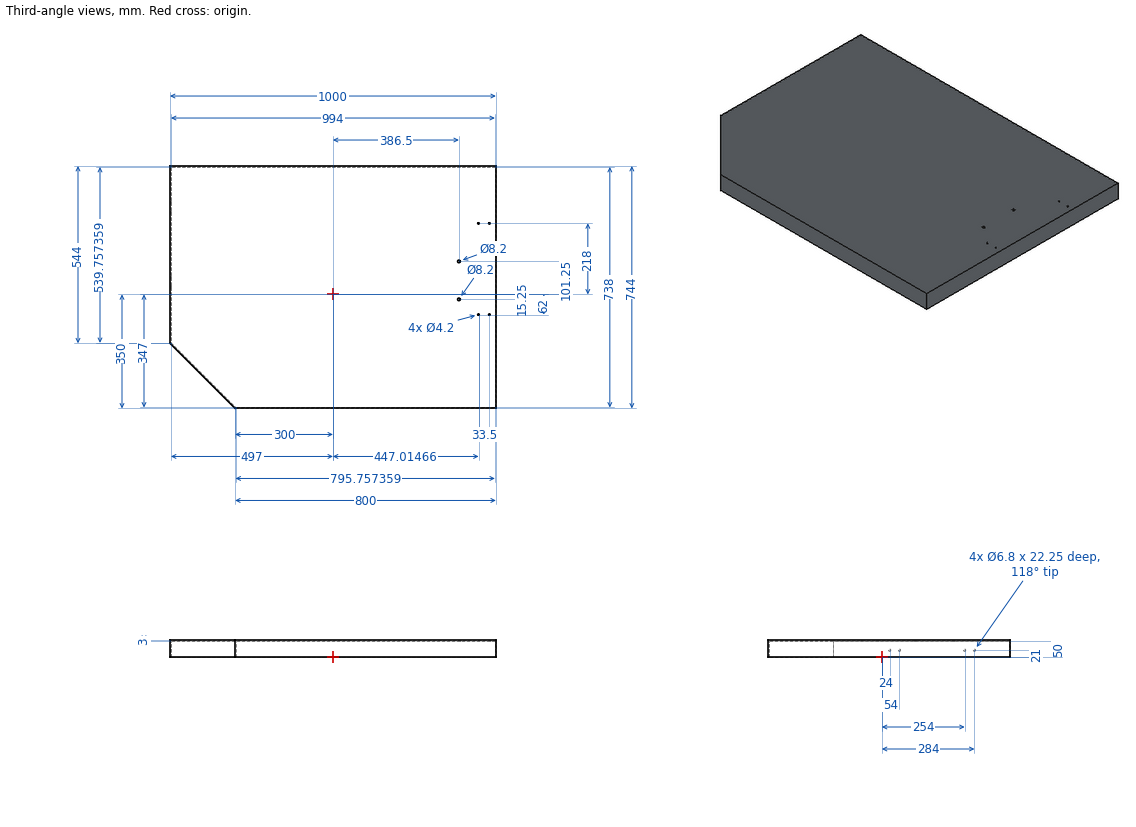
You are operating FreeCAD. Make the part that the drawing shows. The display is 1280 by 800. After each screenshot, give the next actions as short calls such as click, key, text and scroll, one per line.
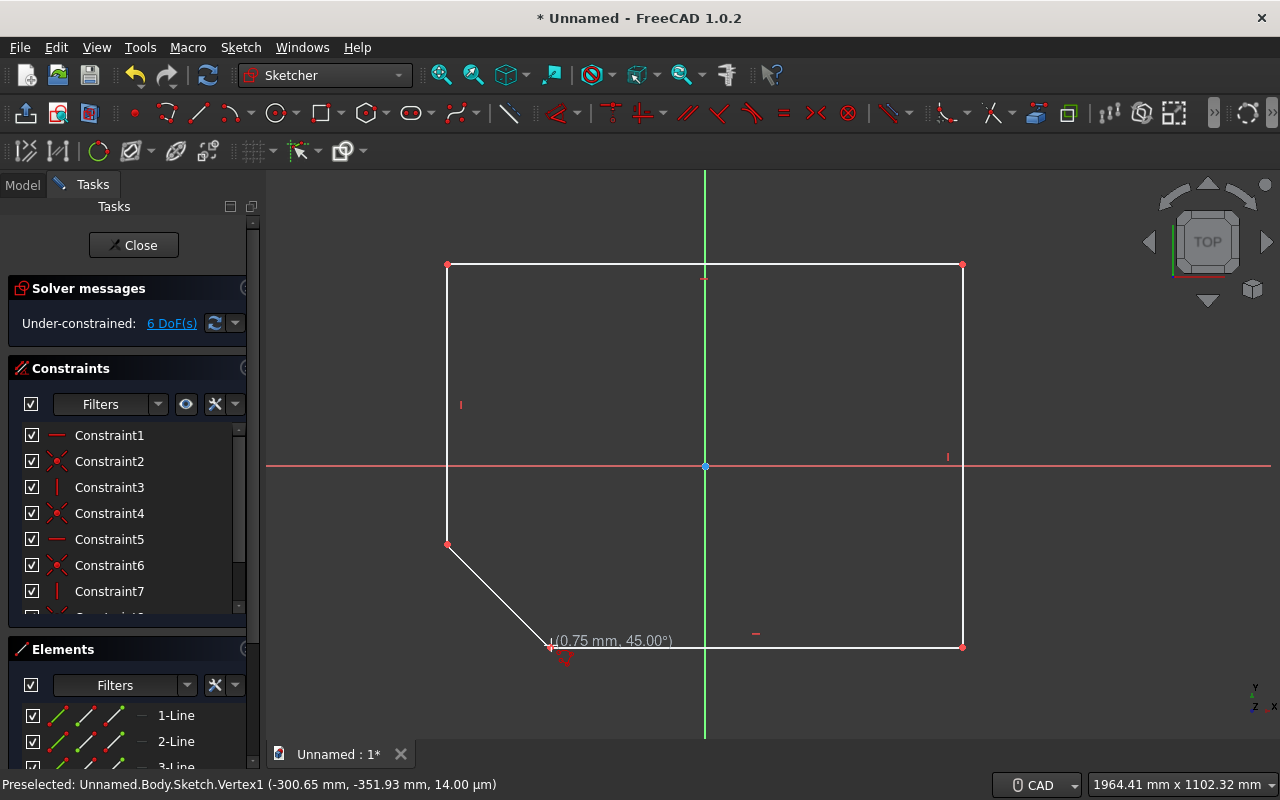
scroll(449, 543, up, 12)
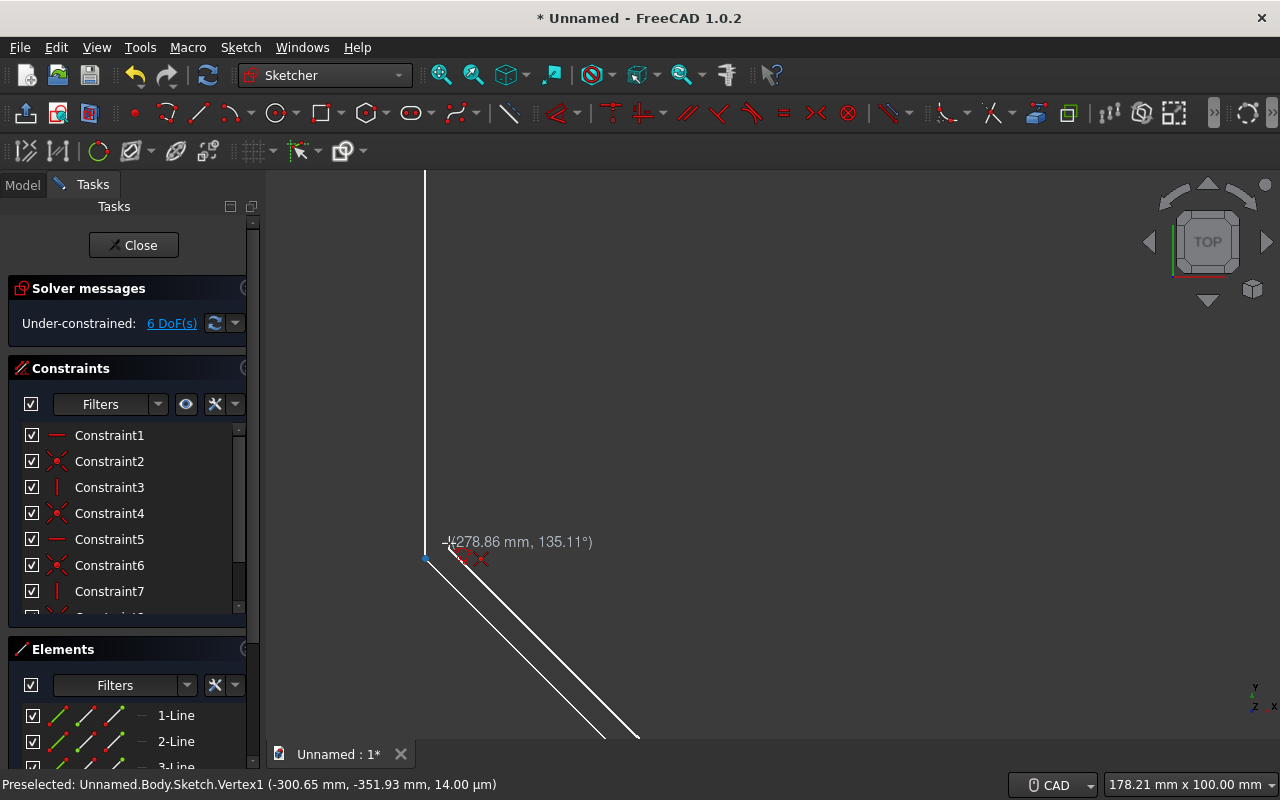
click(443, 538)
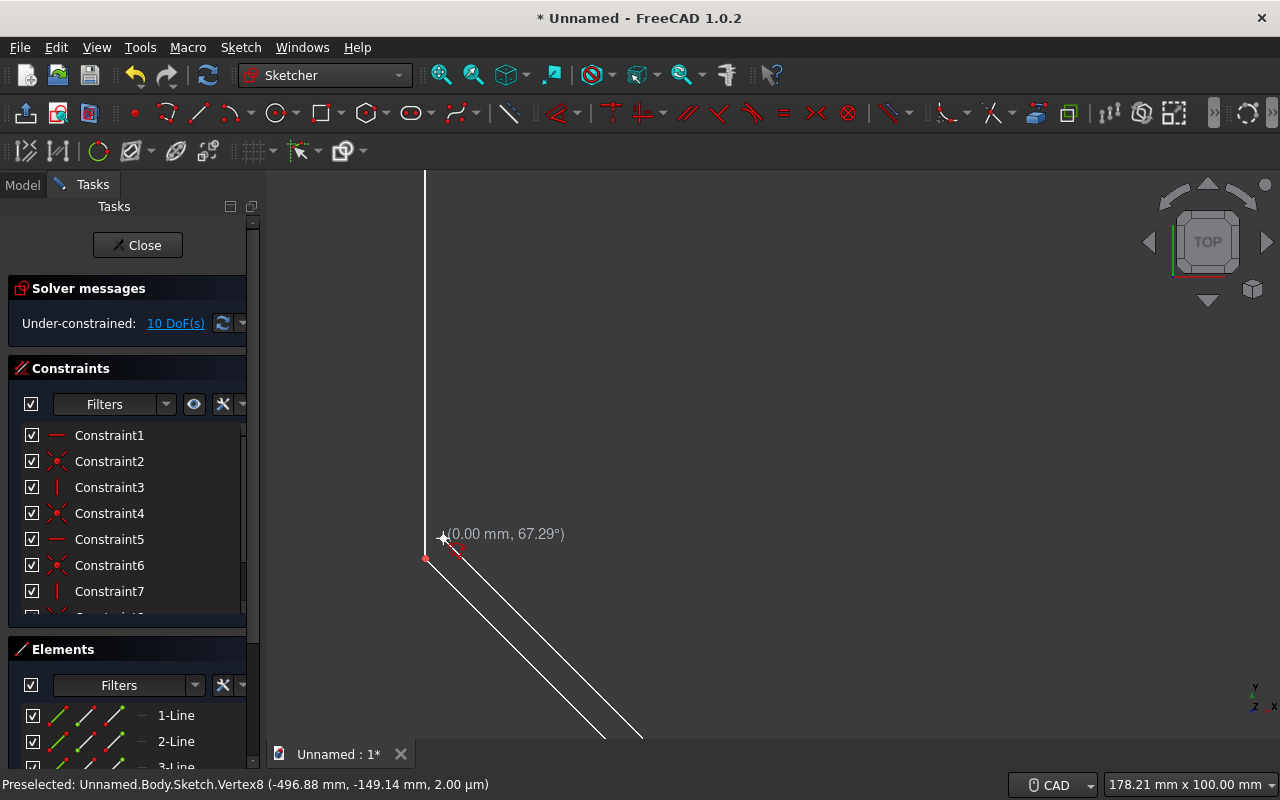
scroll(448, 543, down, 12)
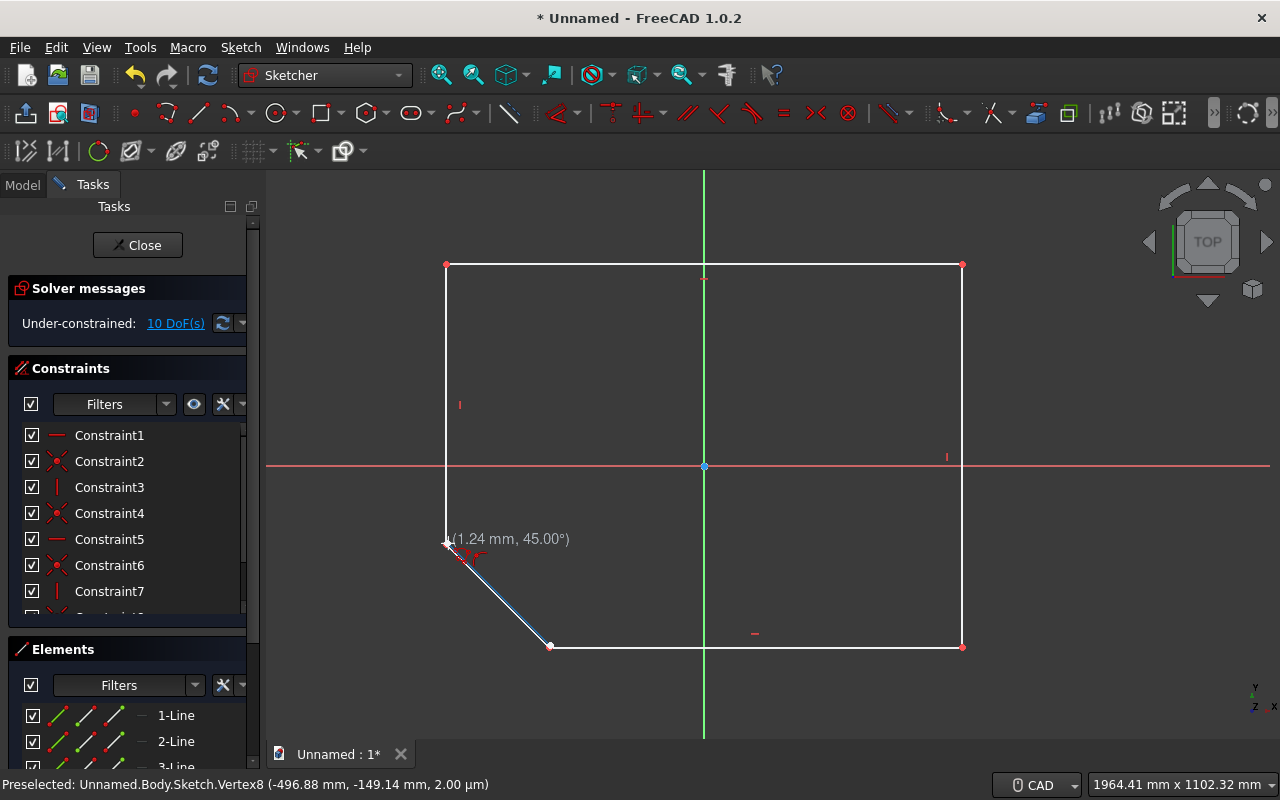
scroll(448, 265, up, 12)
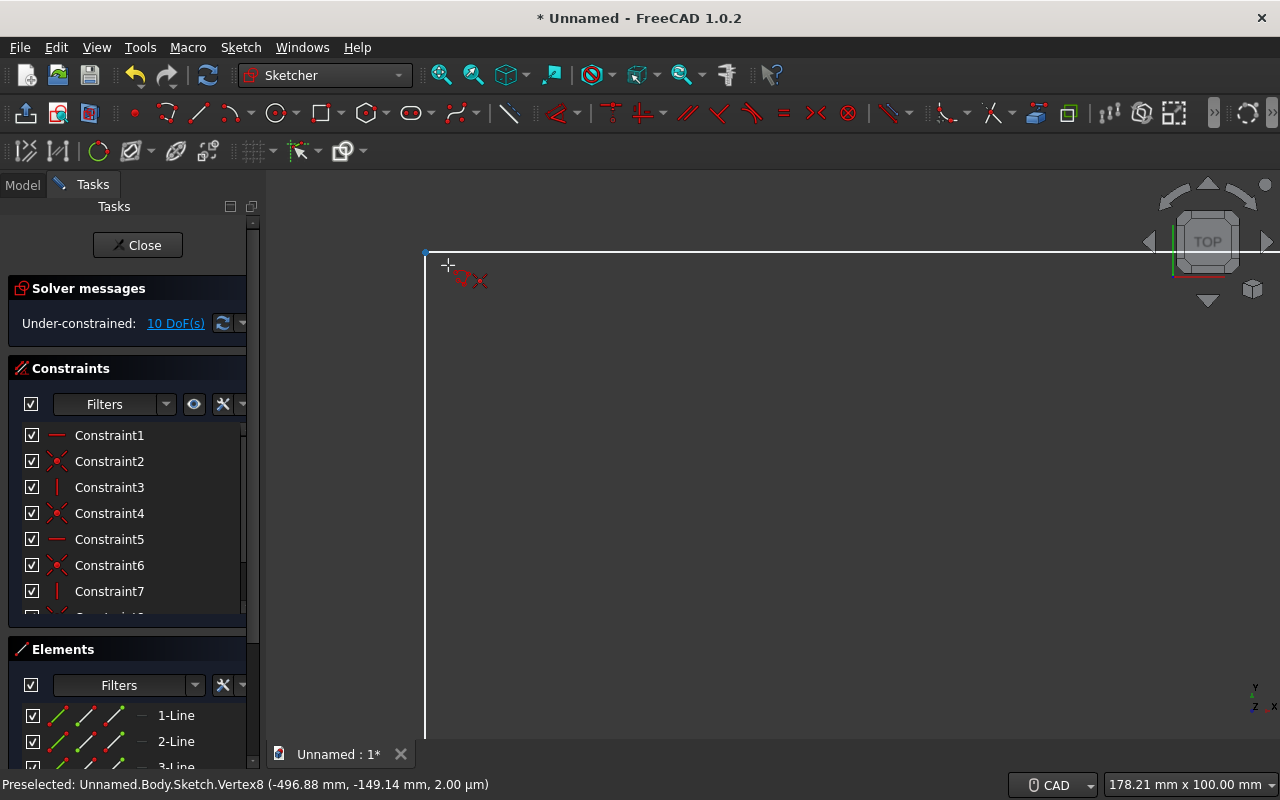
click(443, 258)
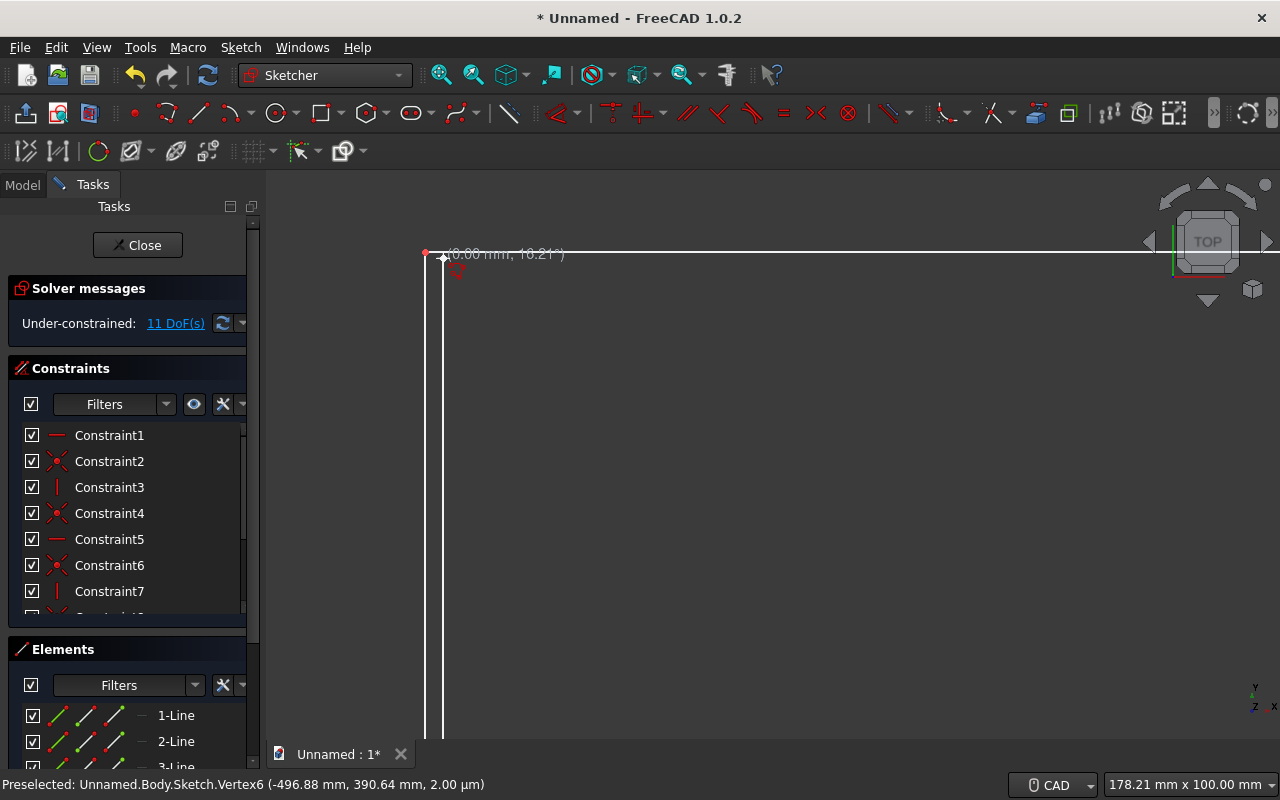
scroll(448, 265, down, 12)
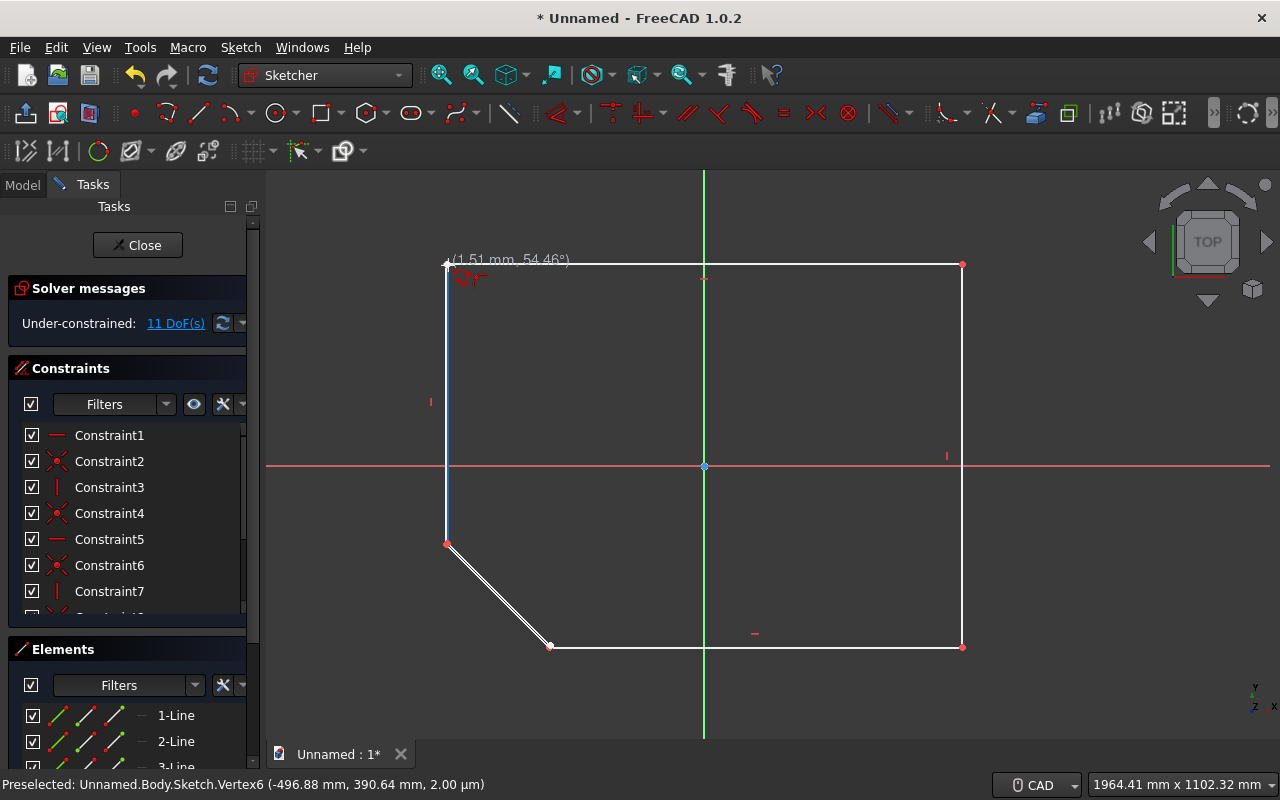
scroll(961, 265, up, 12)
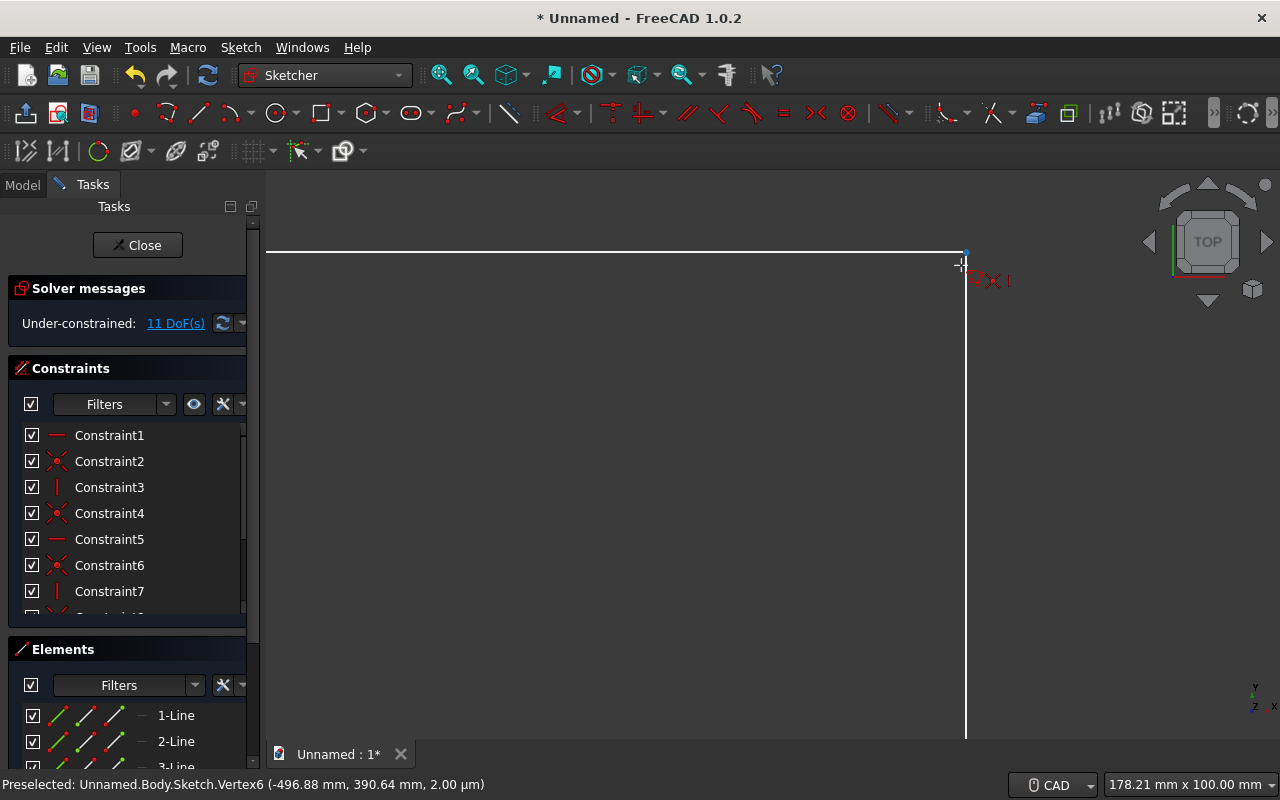
click(952, 258)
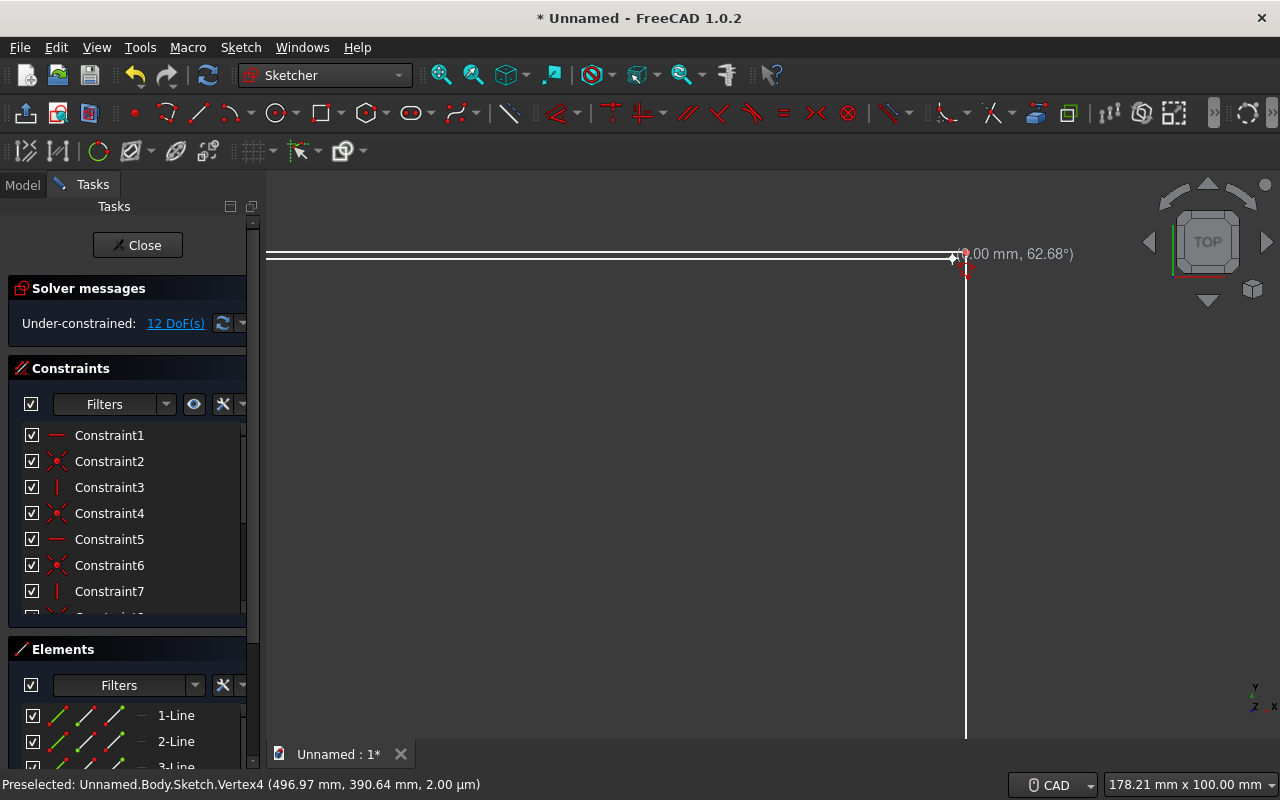
scroll(962, 265, down, 12)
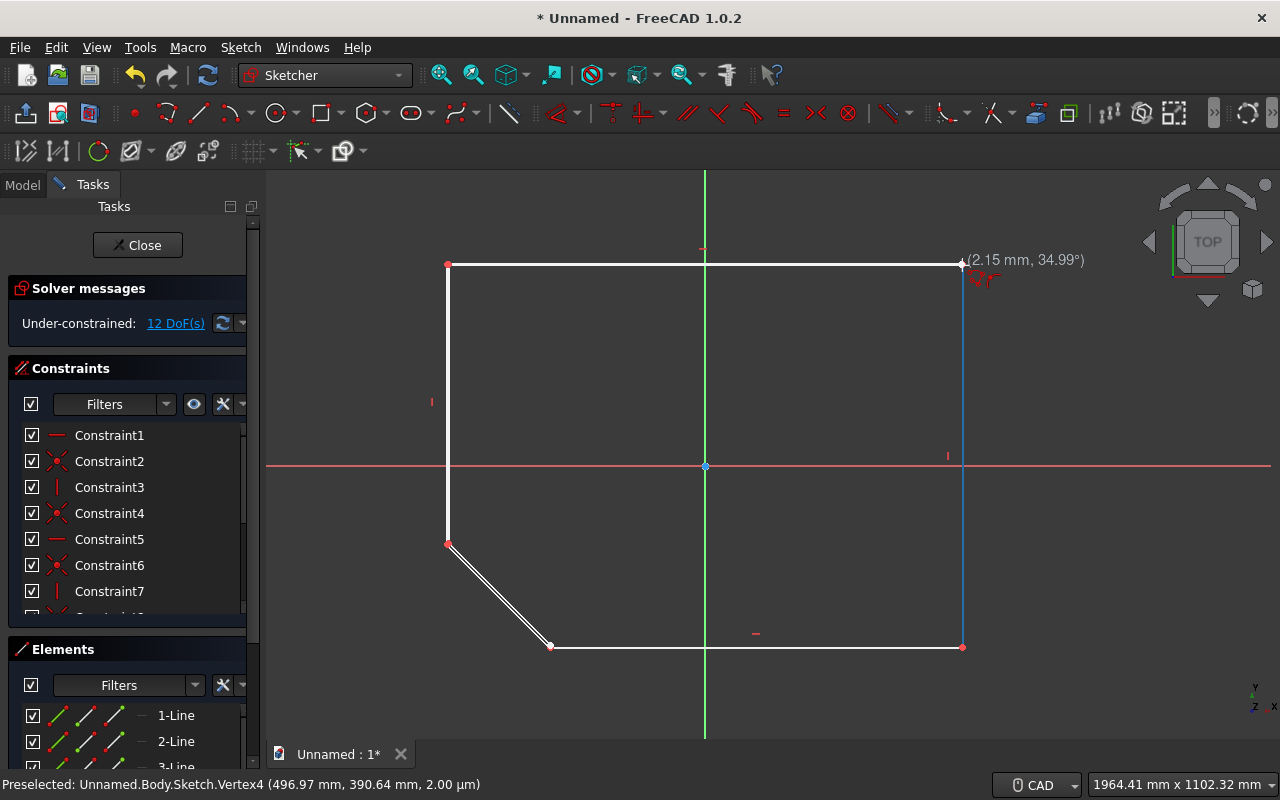
scroll(962, 645, up, 12)